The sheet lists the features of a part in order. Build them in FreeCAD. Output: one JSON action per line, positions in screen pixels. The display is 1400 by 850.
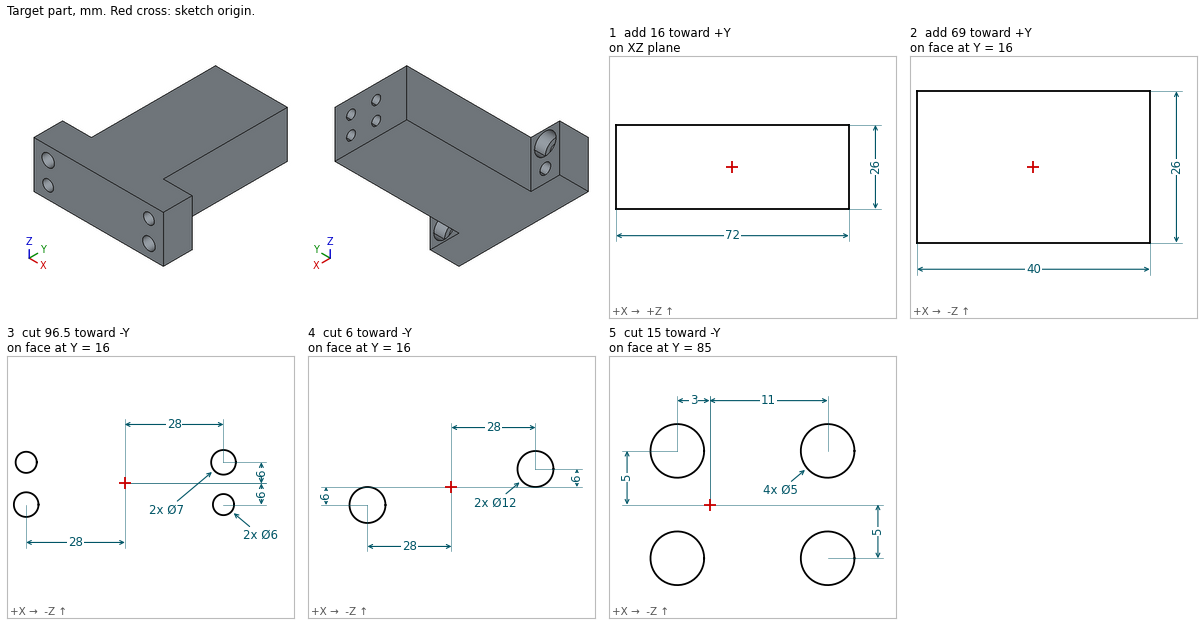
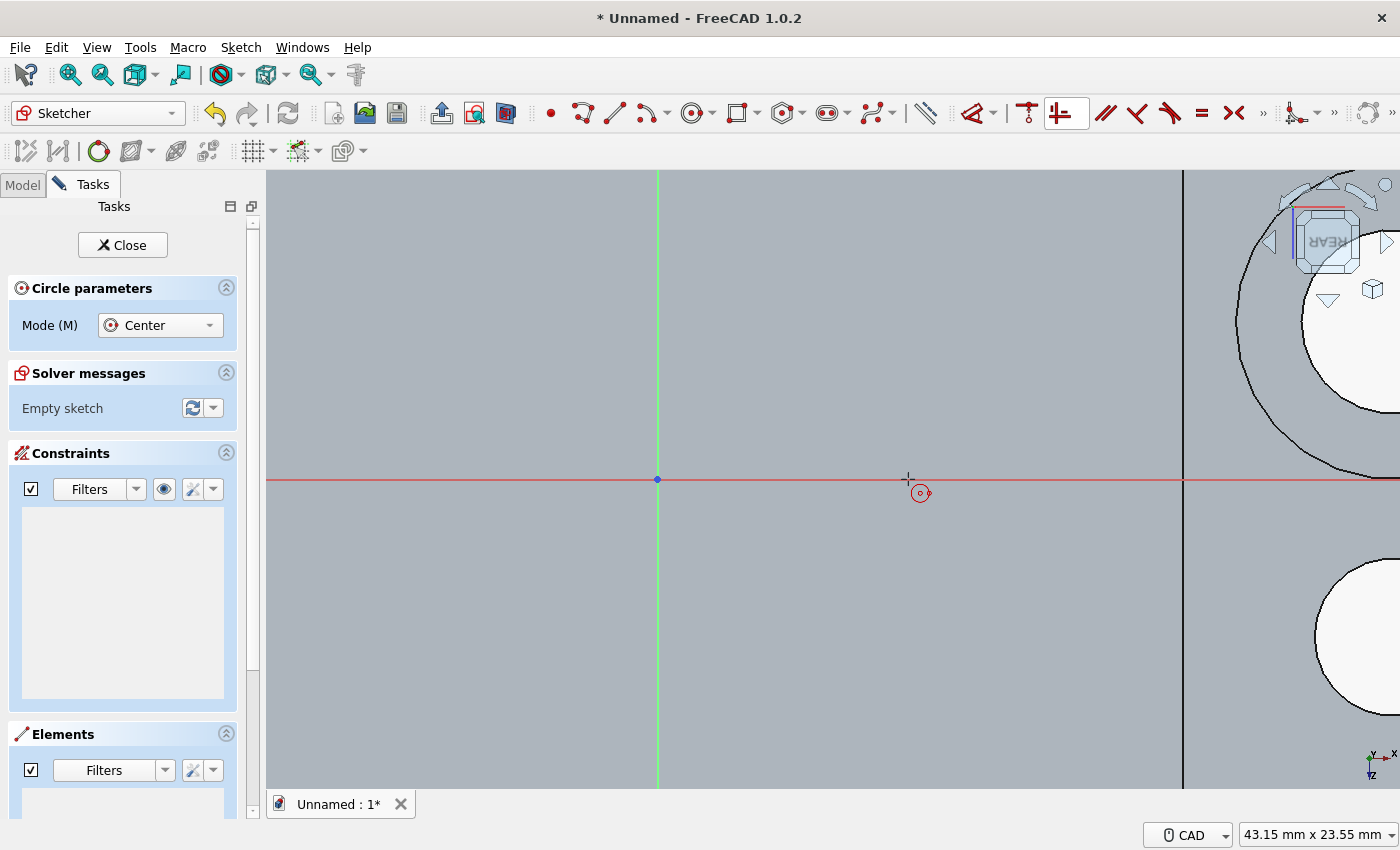
{"action": "left_click", "coordinate": [579, 348]}
{"action": "mouse_move", "coordinate": [625, 302]}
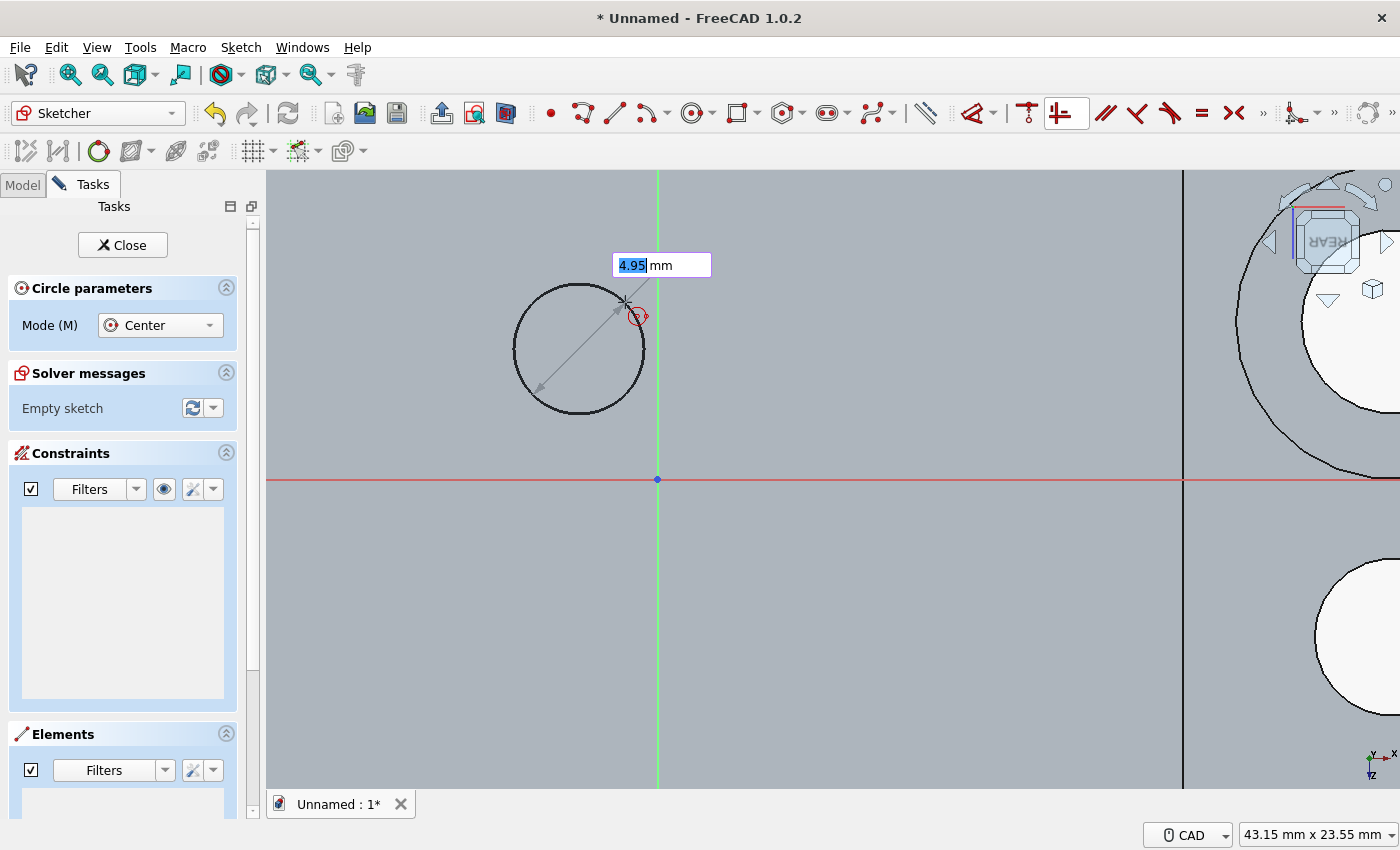
{"action": "type", "text": "5"}
{"action": "key", "text": "Return"}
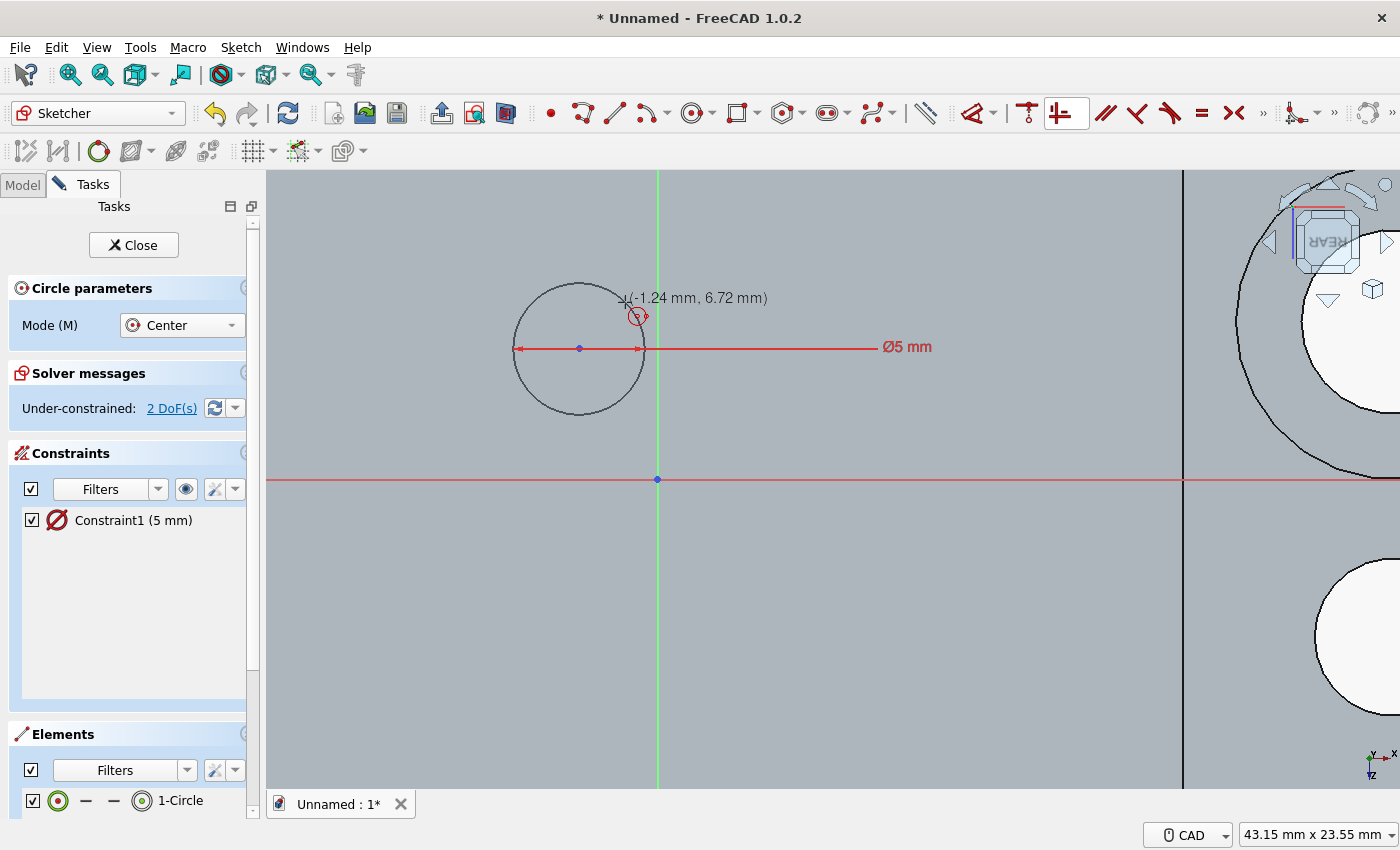
{"action": "left_click", "coordinate": [947, 348]}
{"action": "mouse_move", "coordinate": [993, 302]}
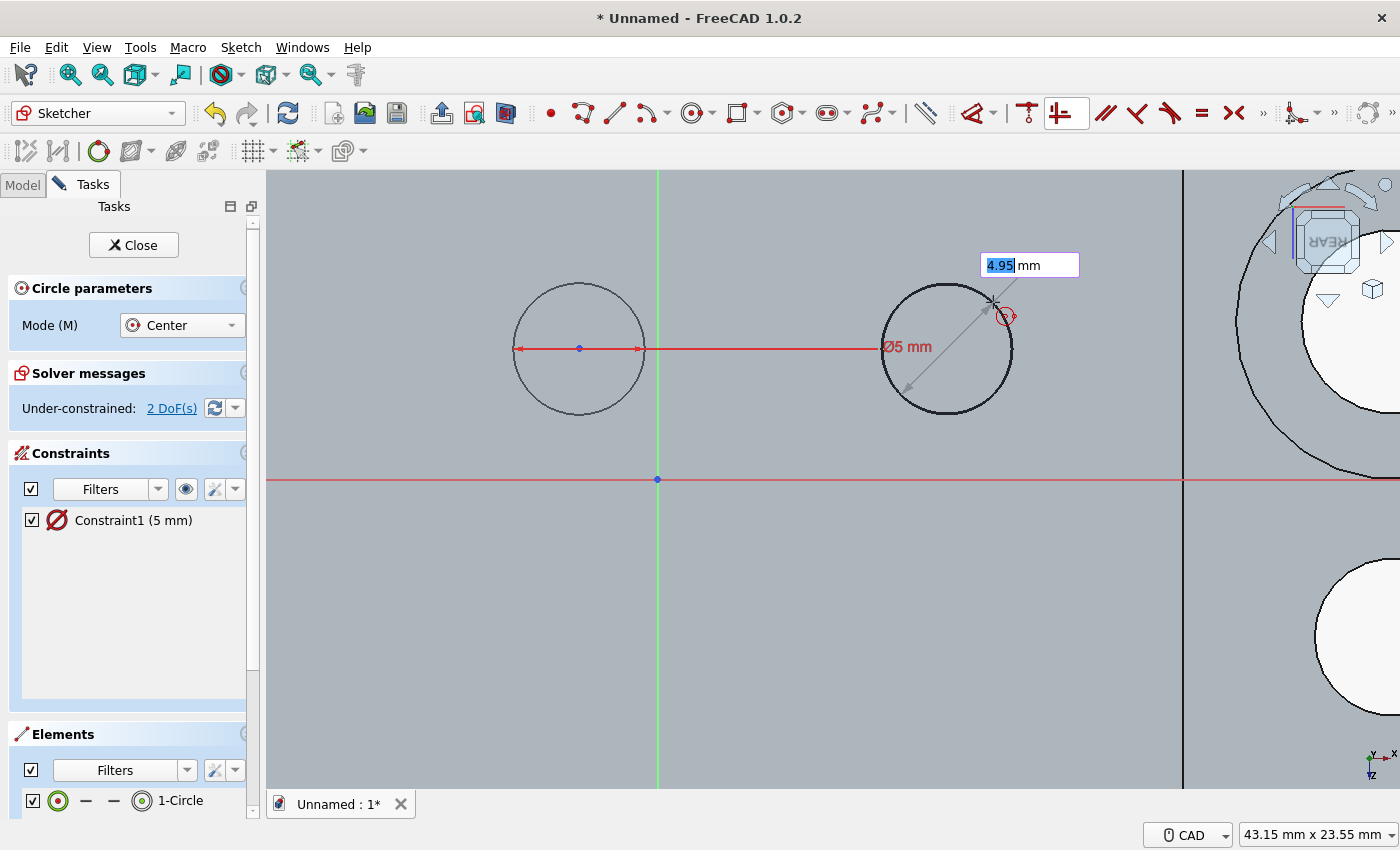
{"action": "type", "text": "5"}
{"action": "key", "text": "Return"}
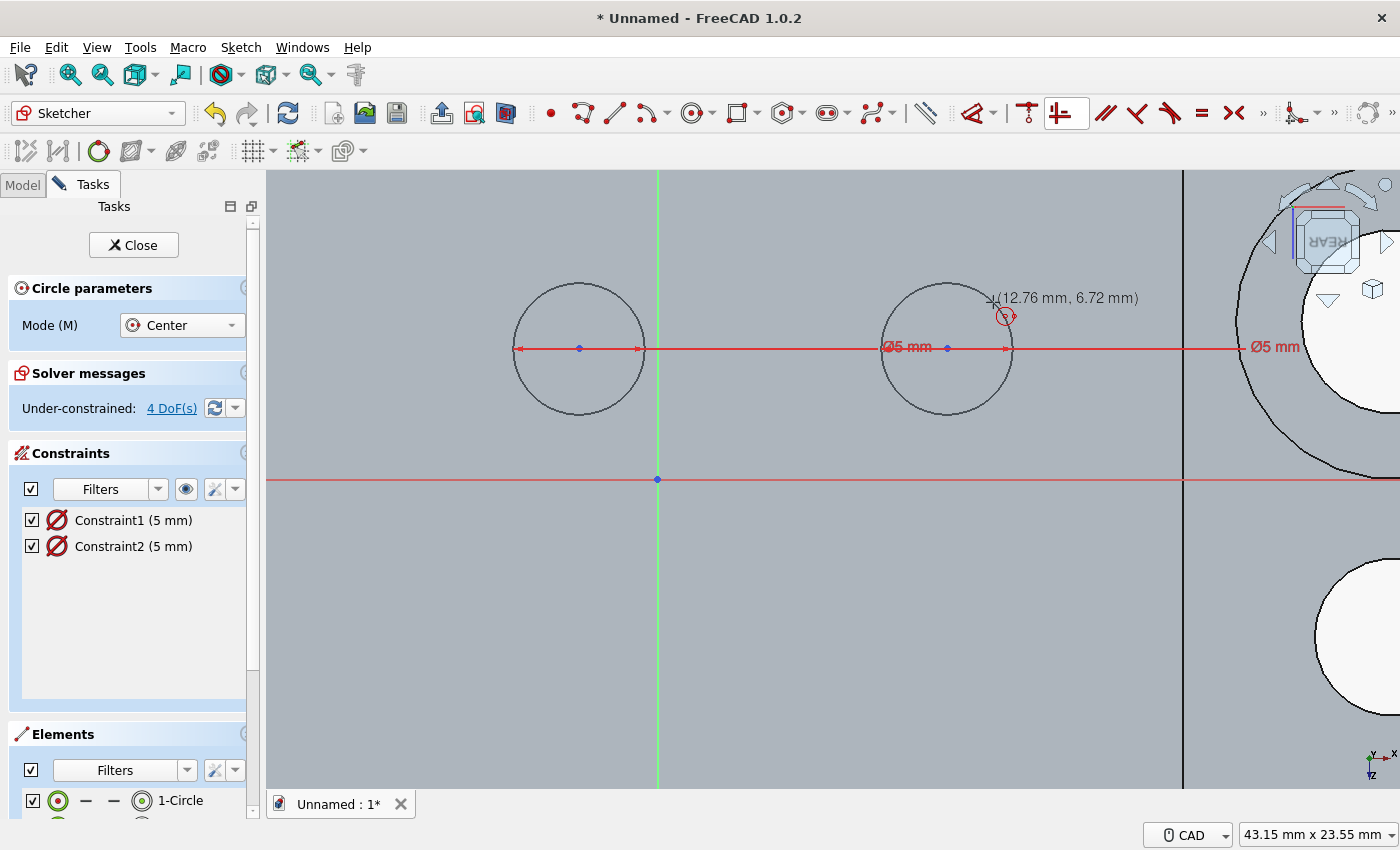
{"action": "left_click", "coordinate": [947, 611]}
{"action": "mouse_move", "coordinate": [993, 564]}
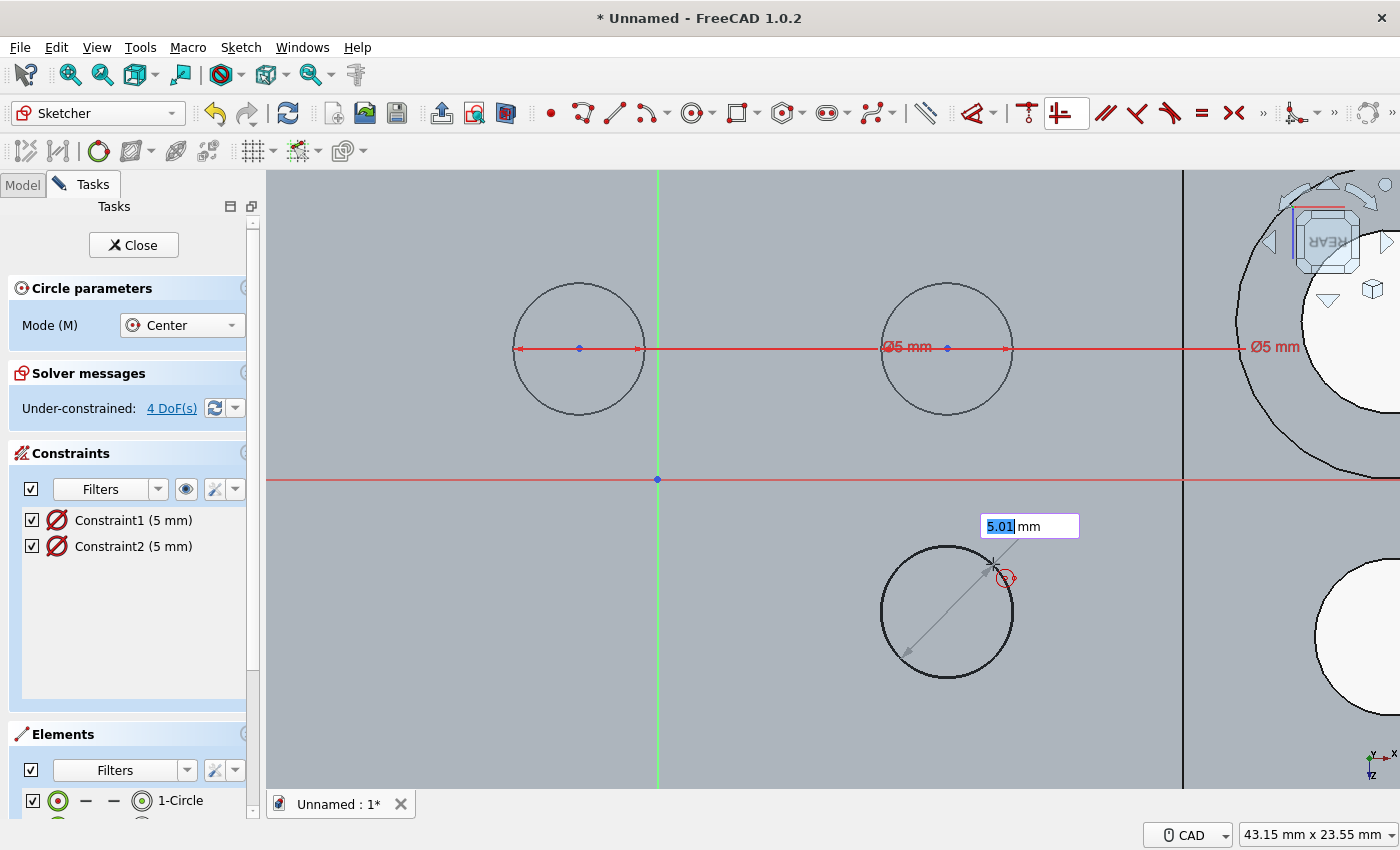
{"action": "type", "text": "5"}
{"action": "key", "text": "Return"}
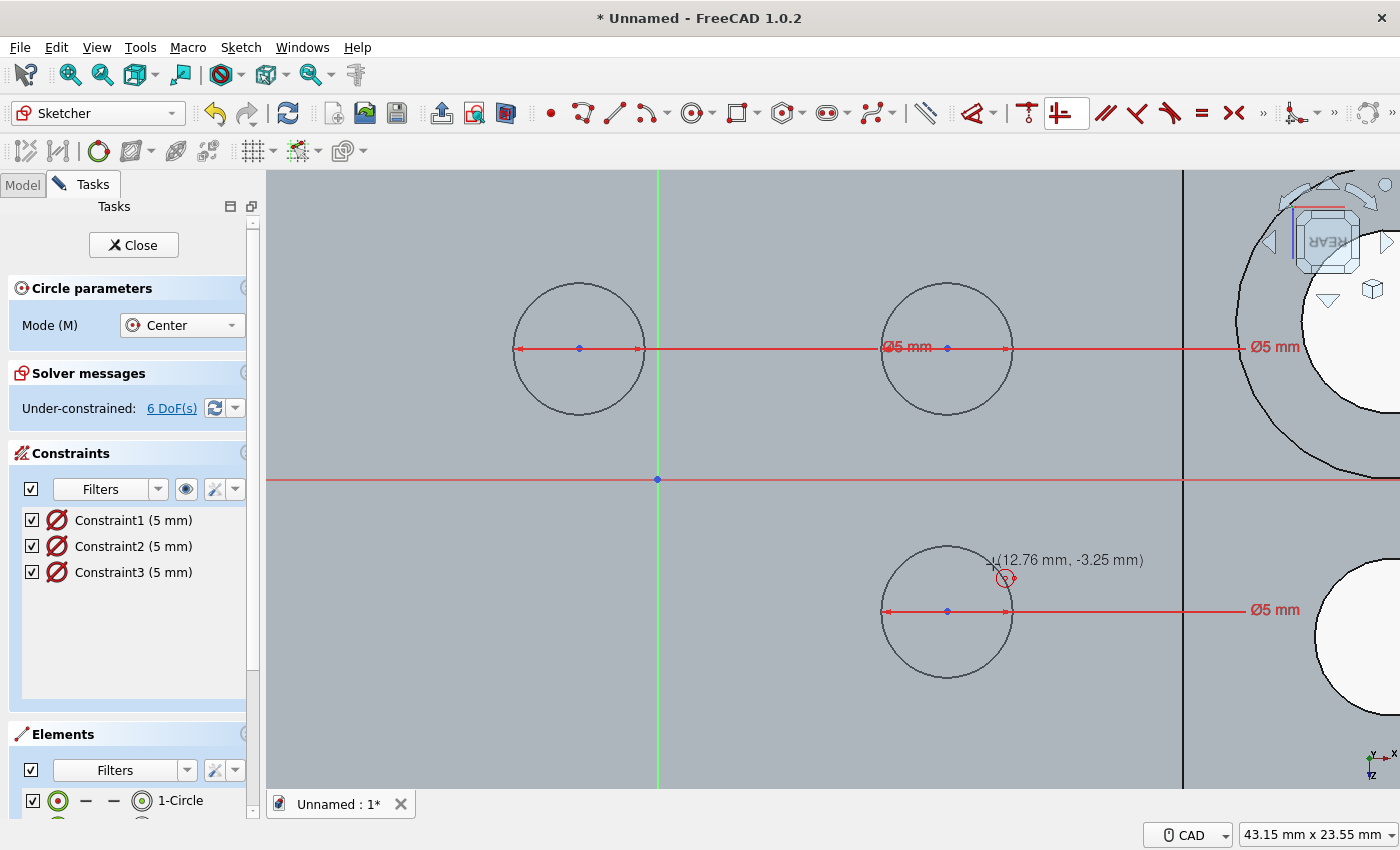
{"action": "left_click", "coordinate": [579, 611]}
{"action": "mouse_move", "coordinate": [625, 564]}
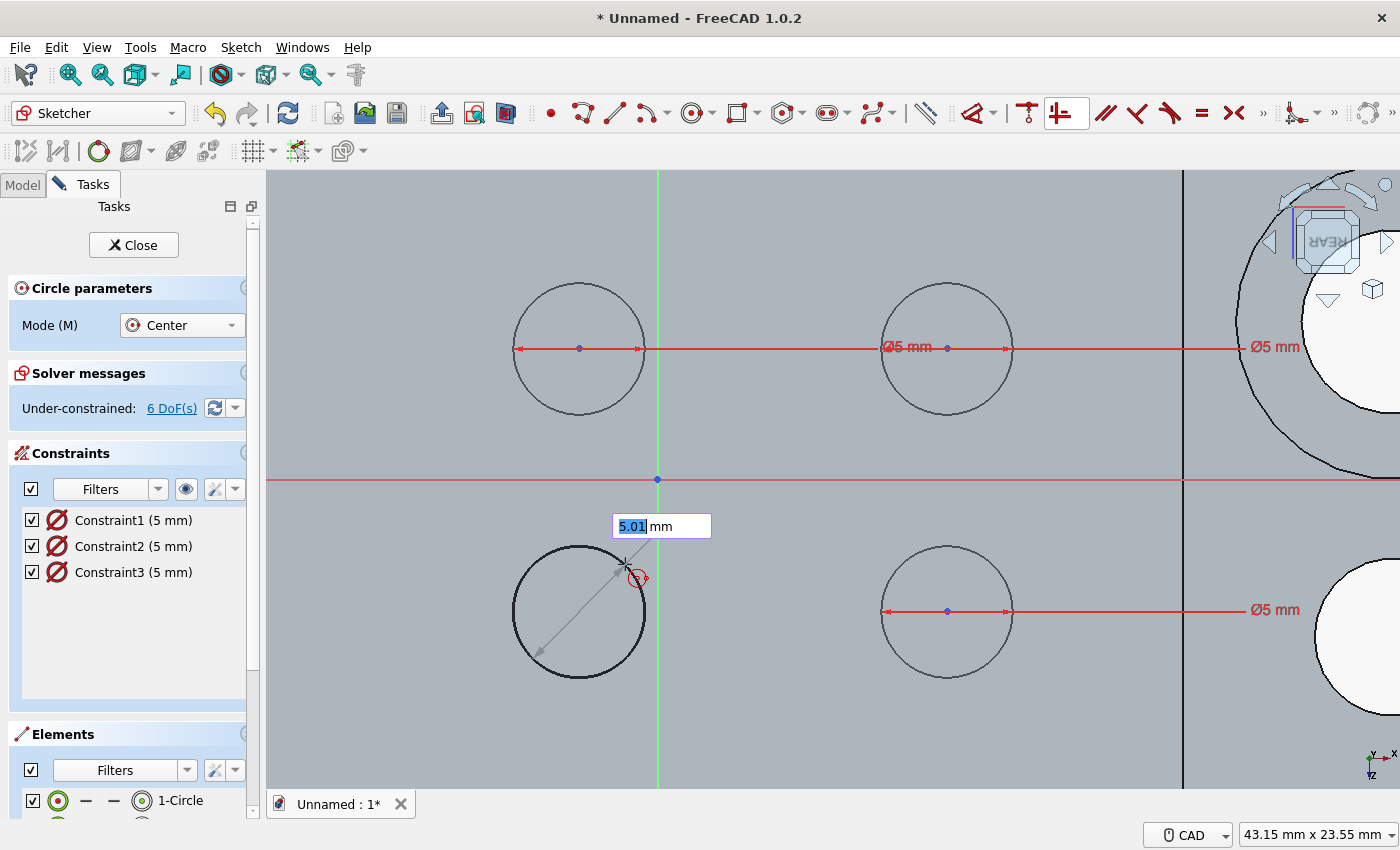
{"action": "type", "text": "5"}
{"action": "key", "text": "Return"}
{"action": "key", "text": "Escape"}